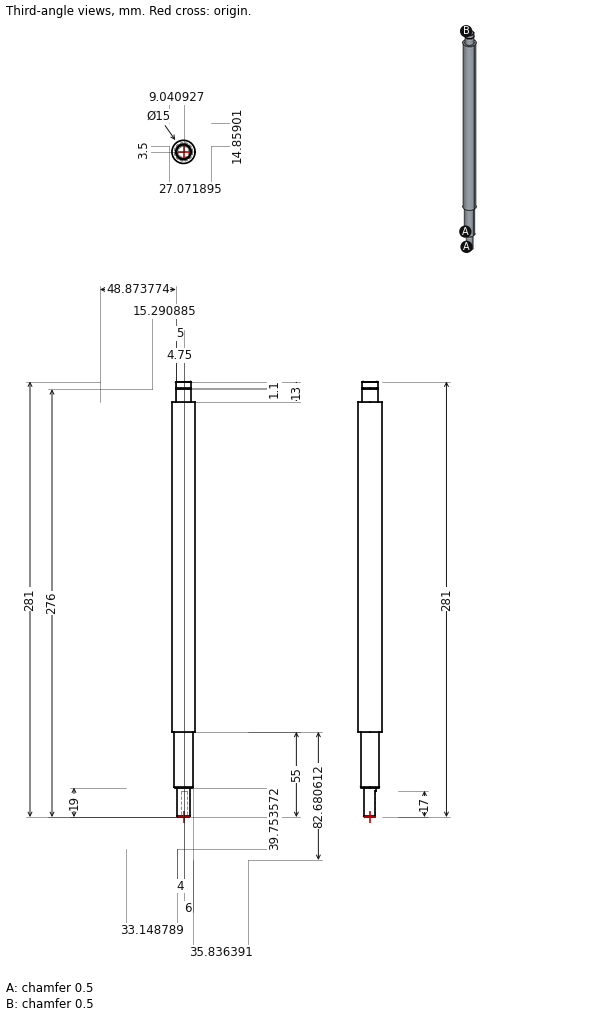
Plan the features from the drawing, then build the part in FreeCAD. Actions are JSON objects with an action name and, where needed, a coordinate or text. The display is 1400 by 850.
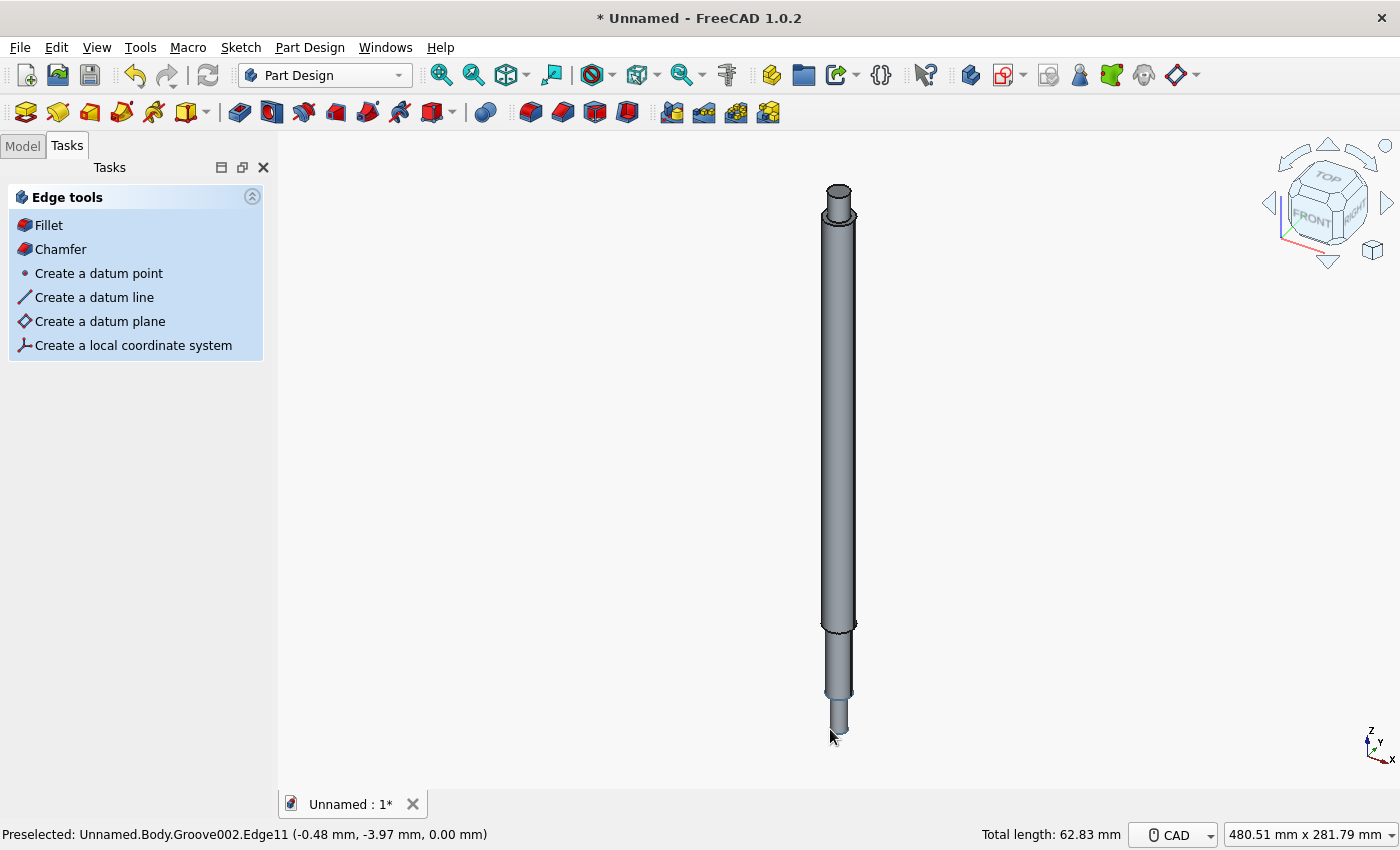
{"action": "left_click", "coordinate": [564, 112]}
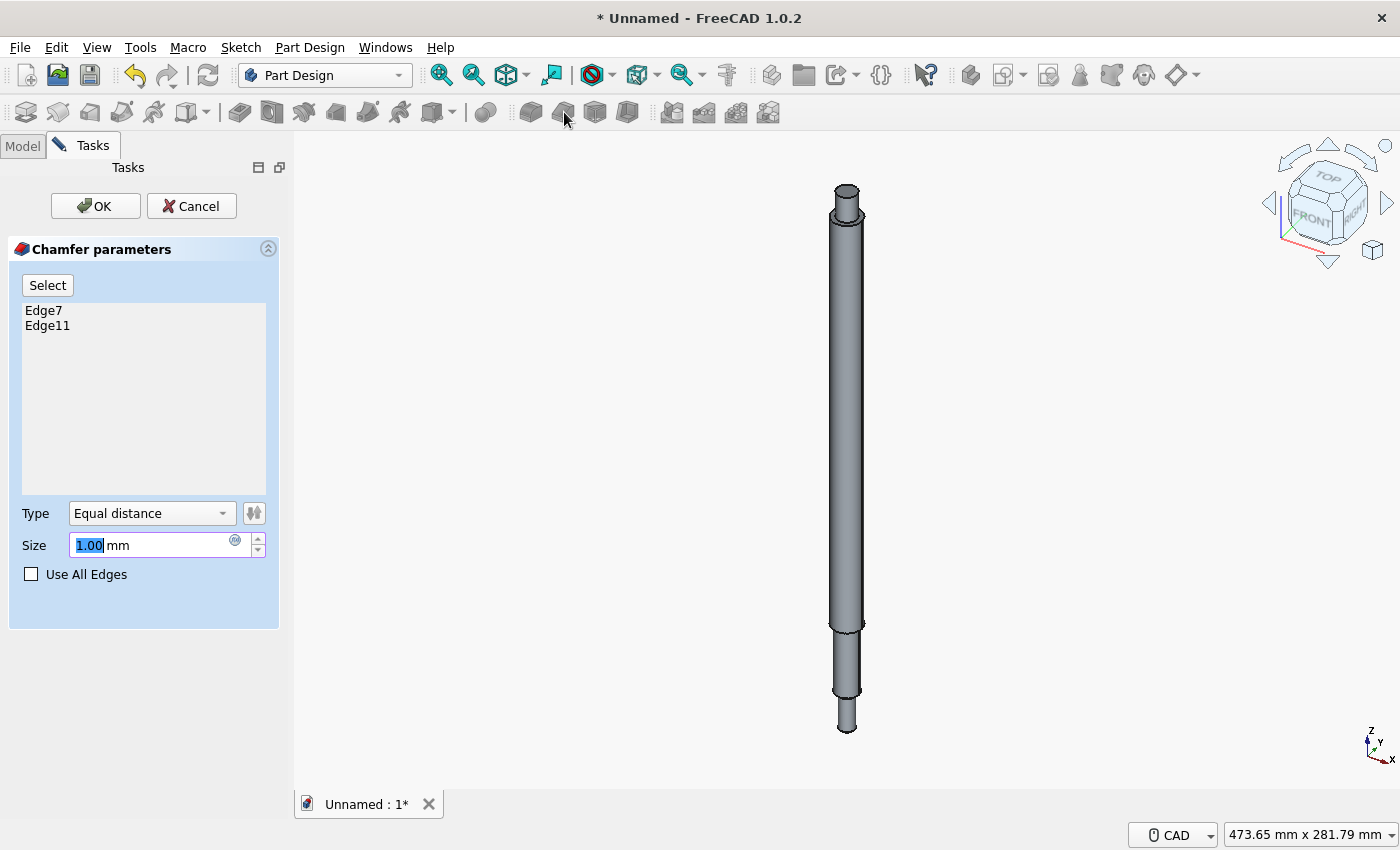
{"action": "type", "text": "0.5"}
{"action": "key", "text": "Tab"}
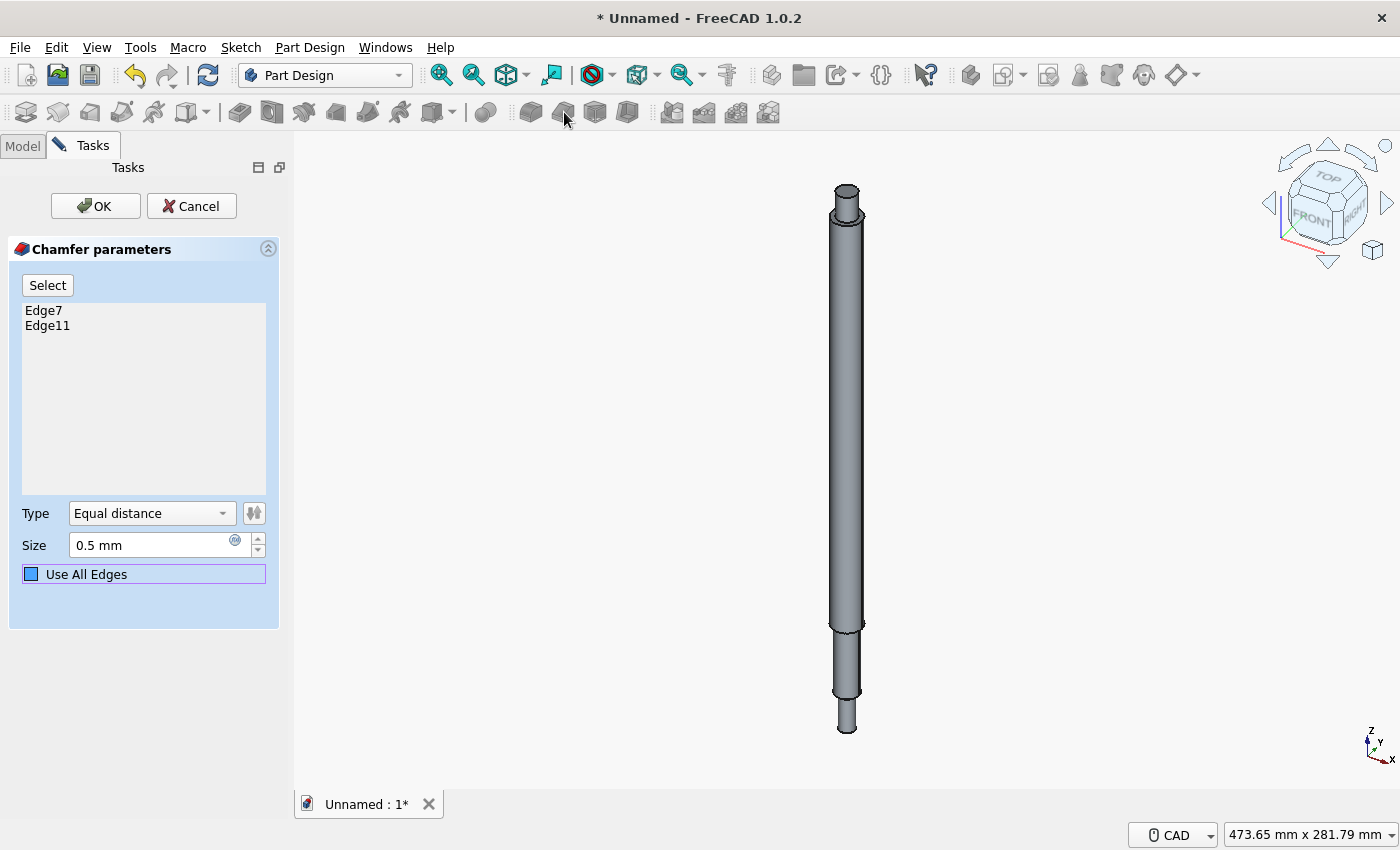
{"action": "left_click", "coordinate": [96, 206]}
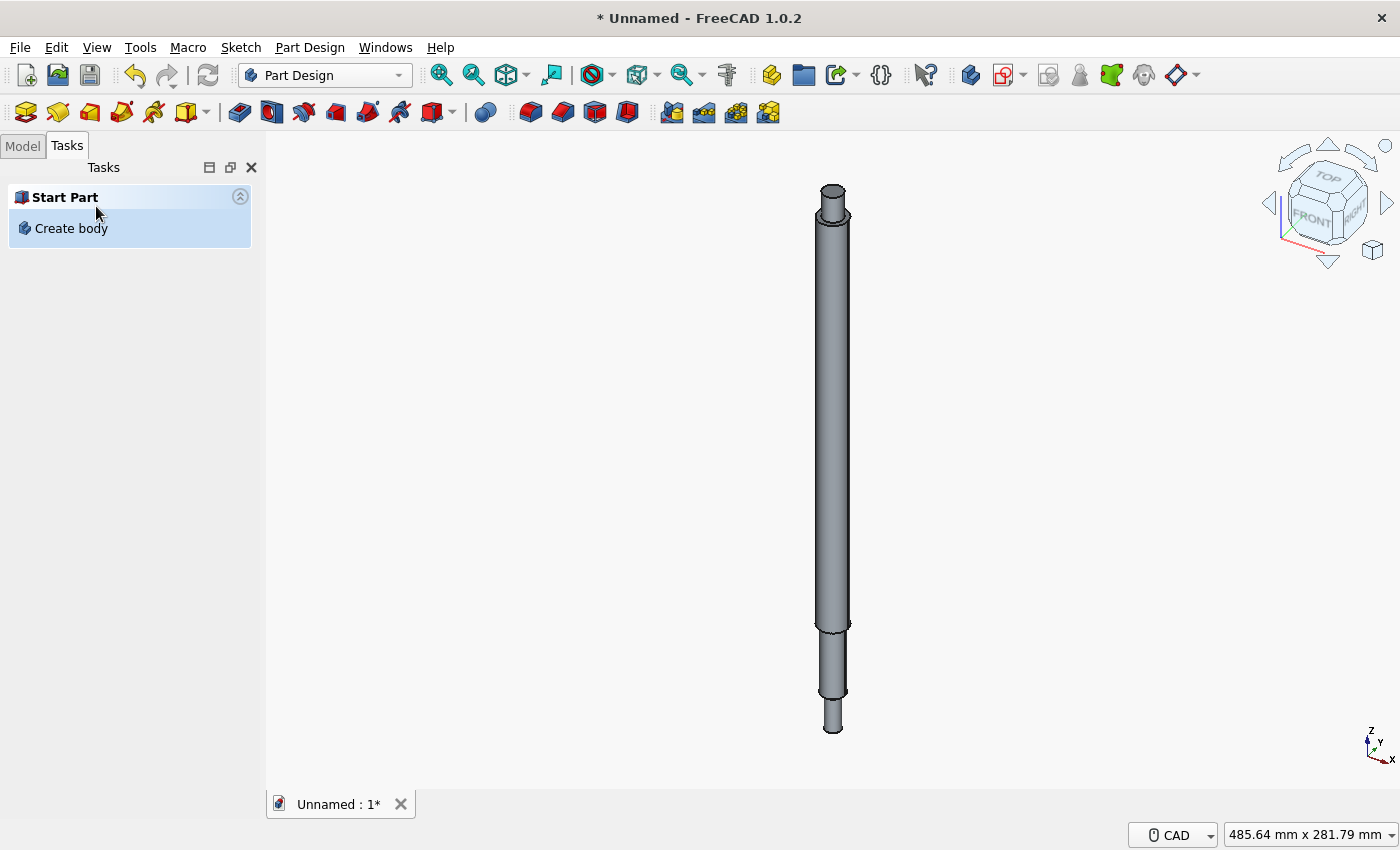
{"action": "left_click", "coordinate": [1004, 76]}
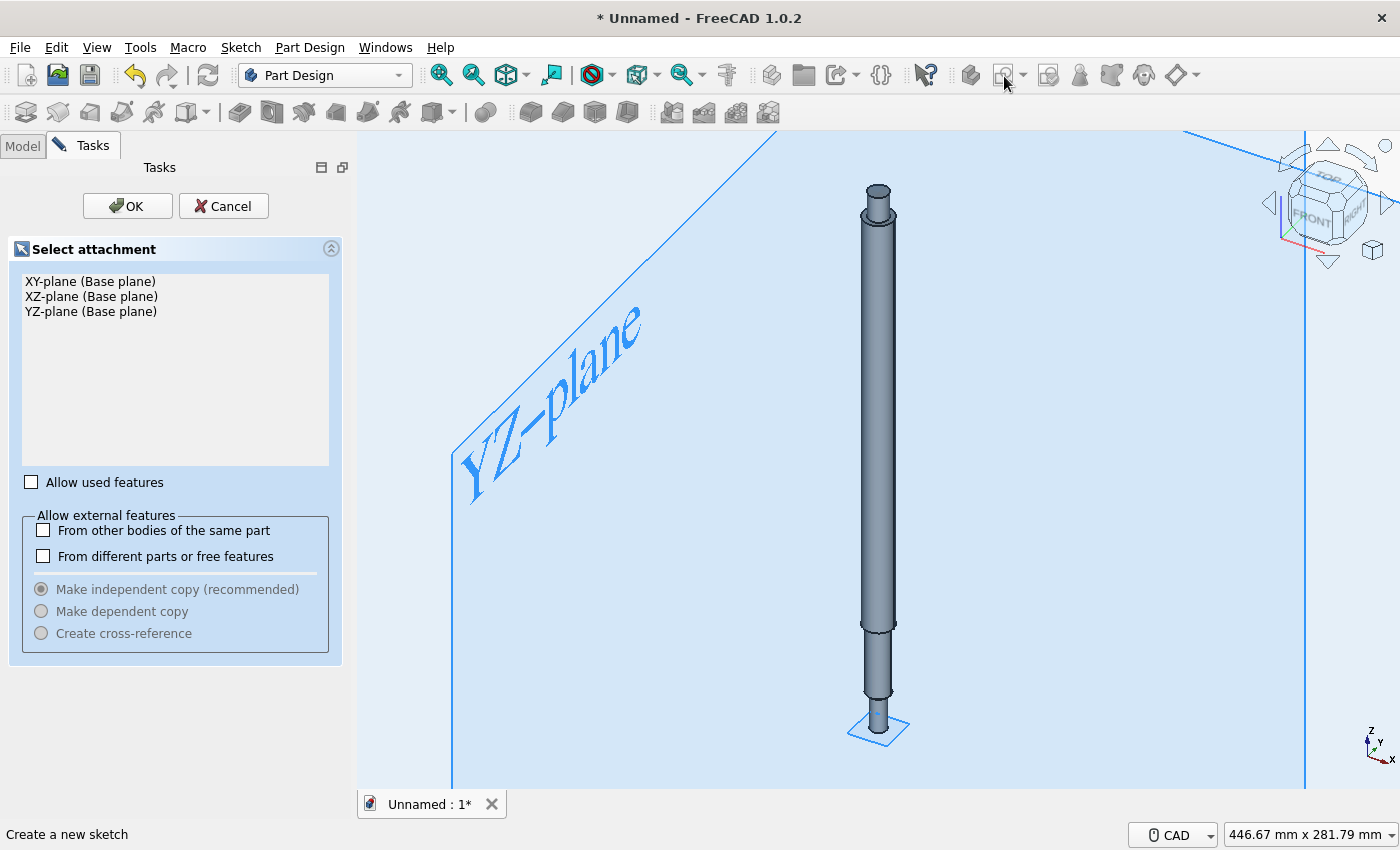
{"action": "left_click", "coordinate": [82, 296]}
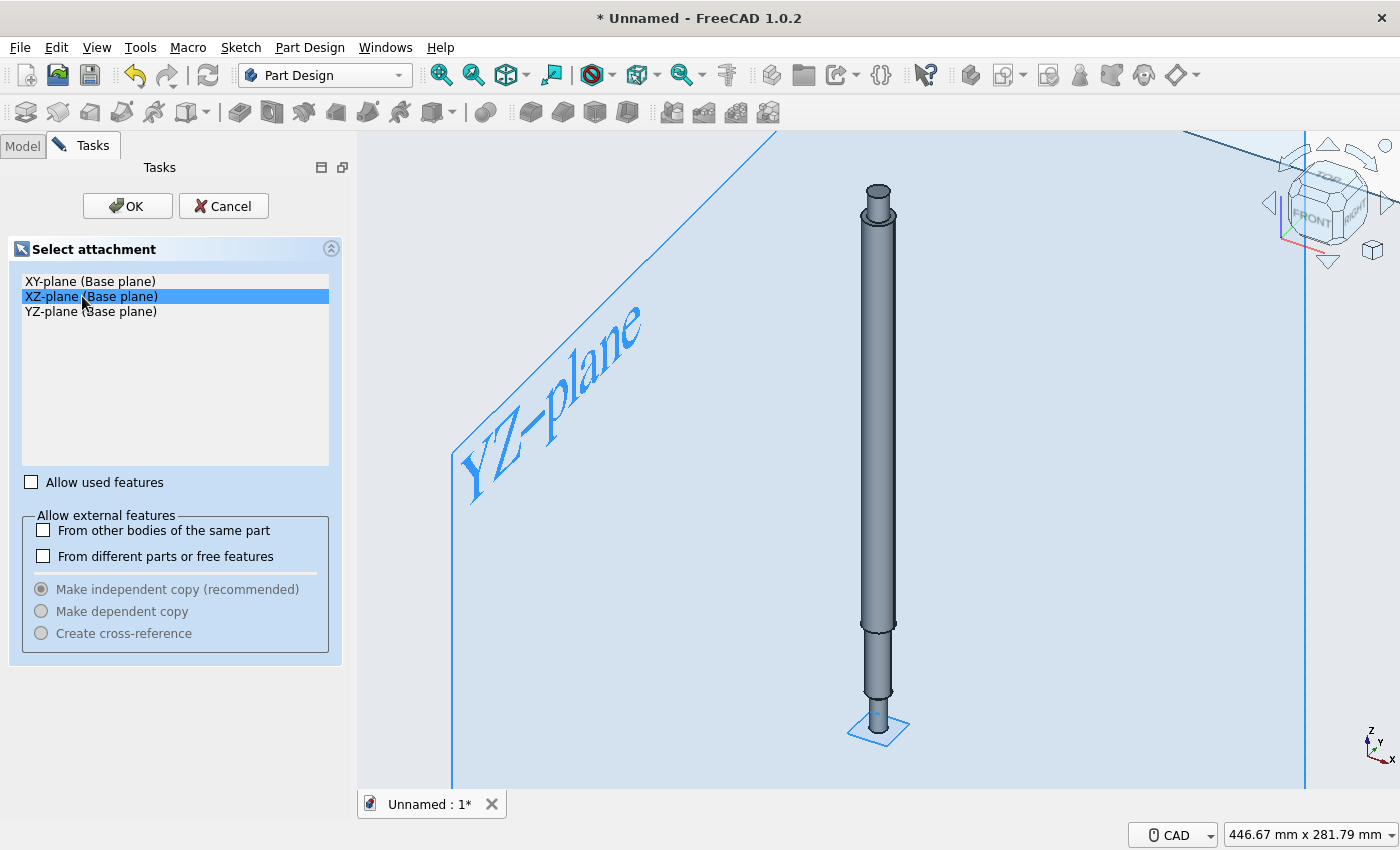
{"action": "left_click", "coordinate": [128, 206]}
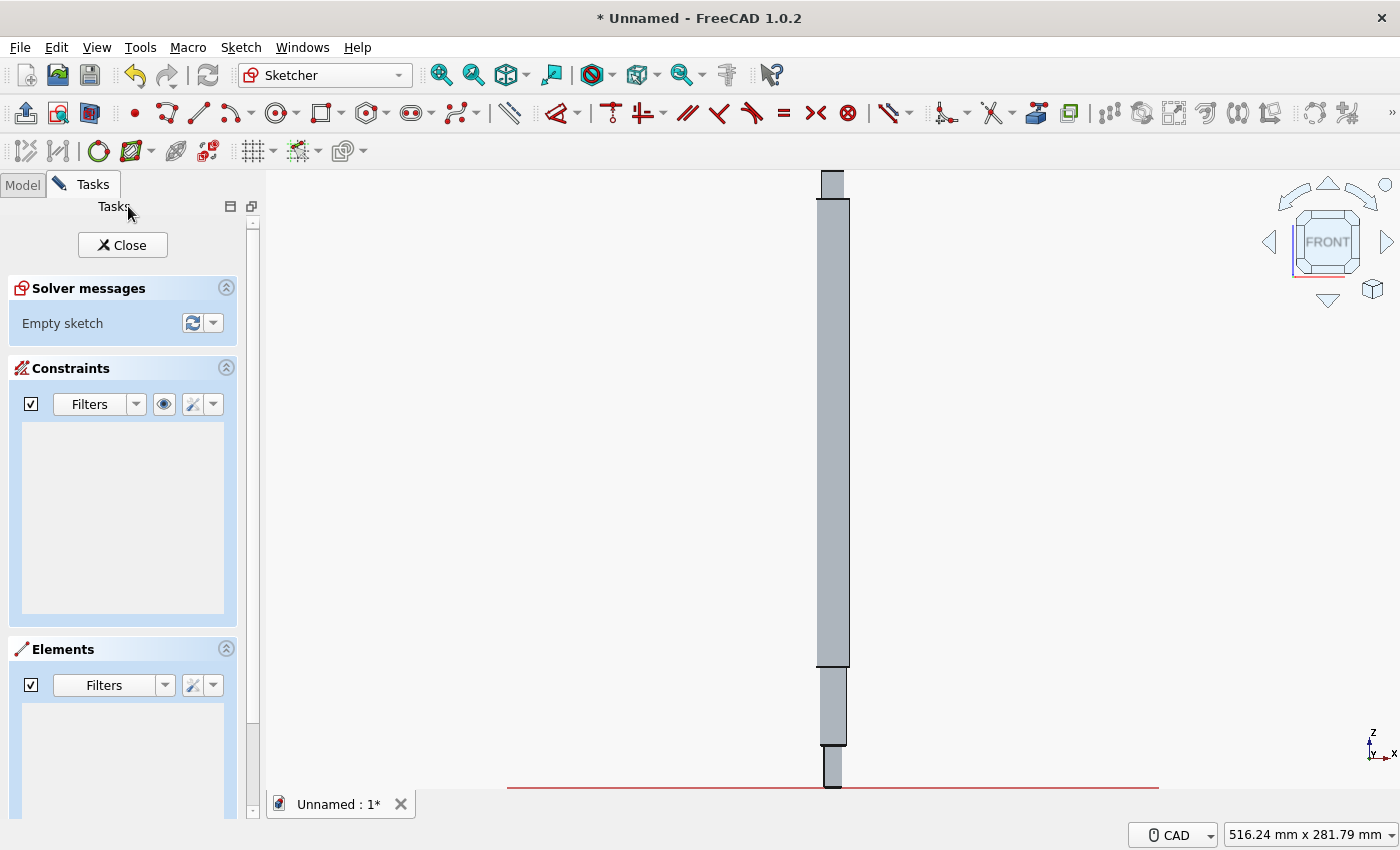
{"action": "left_click", "coordinate": [90, 114]}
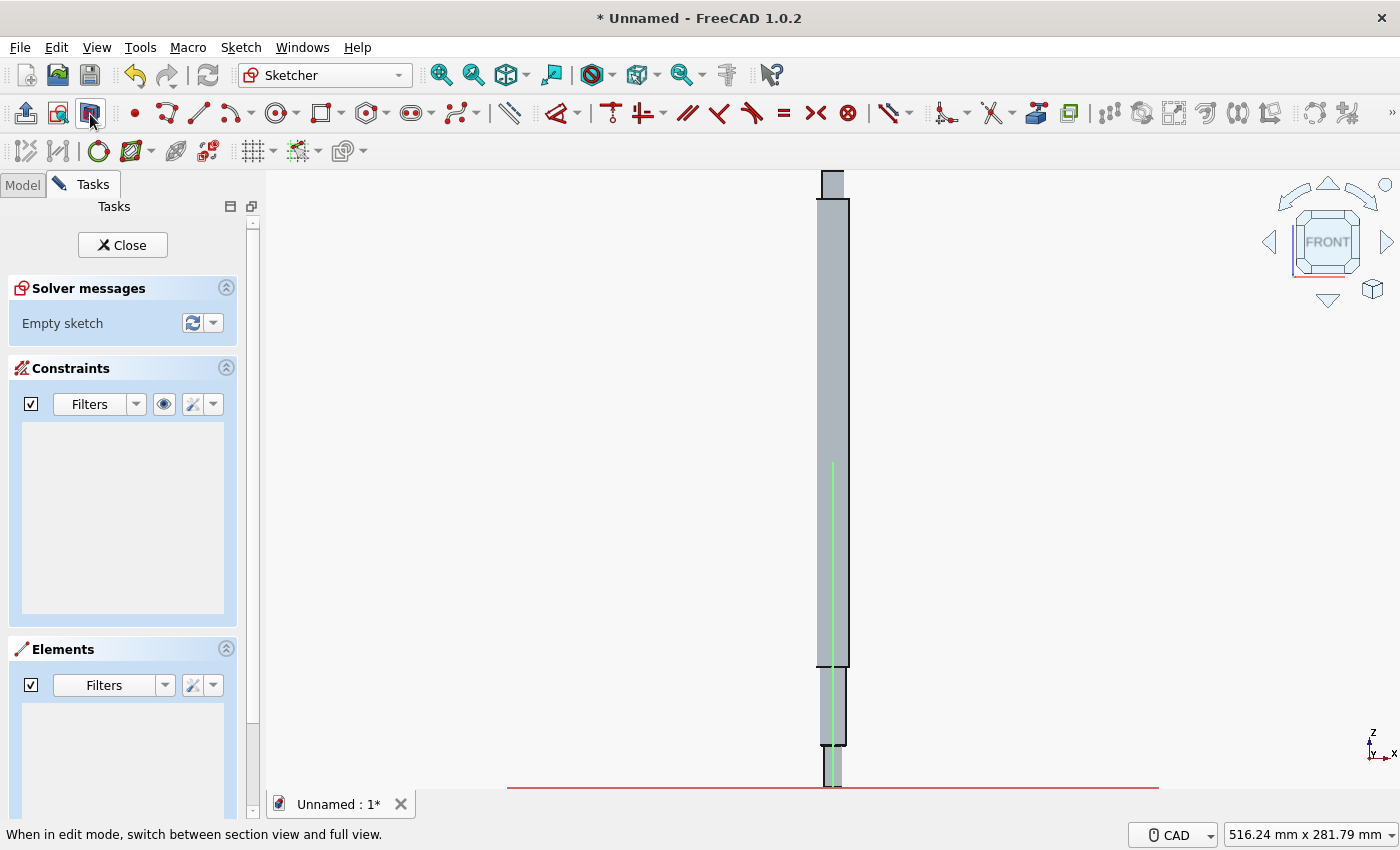
{"action": "scroll", "coordinate": [764, 480], "scroll_direction": "down", "scroll_amount": 5}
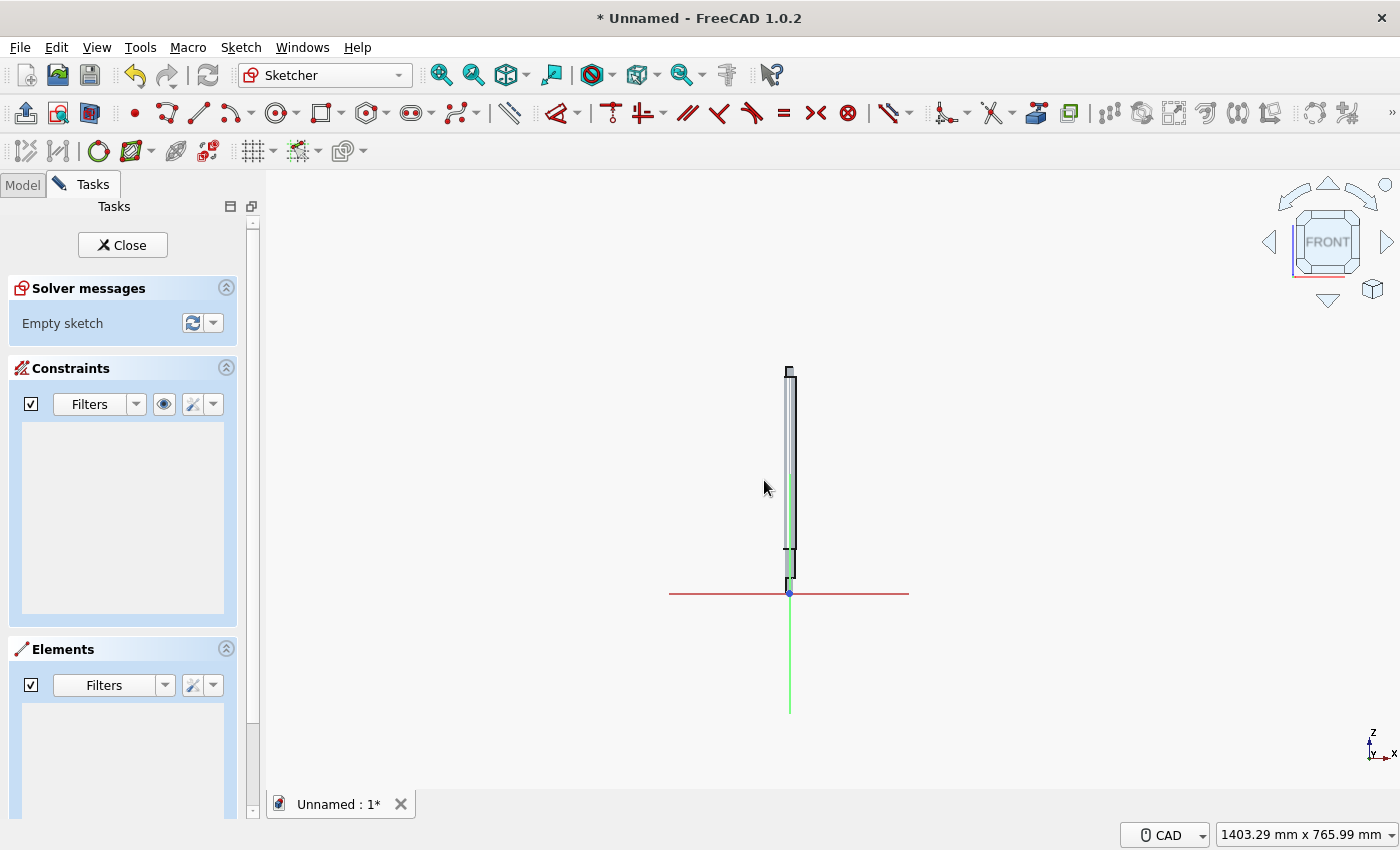
{"action": "scroll", "coordinate": [780, 364], "scroll_direction": "up", "scroll_amount": 15}